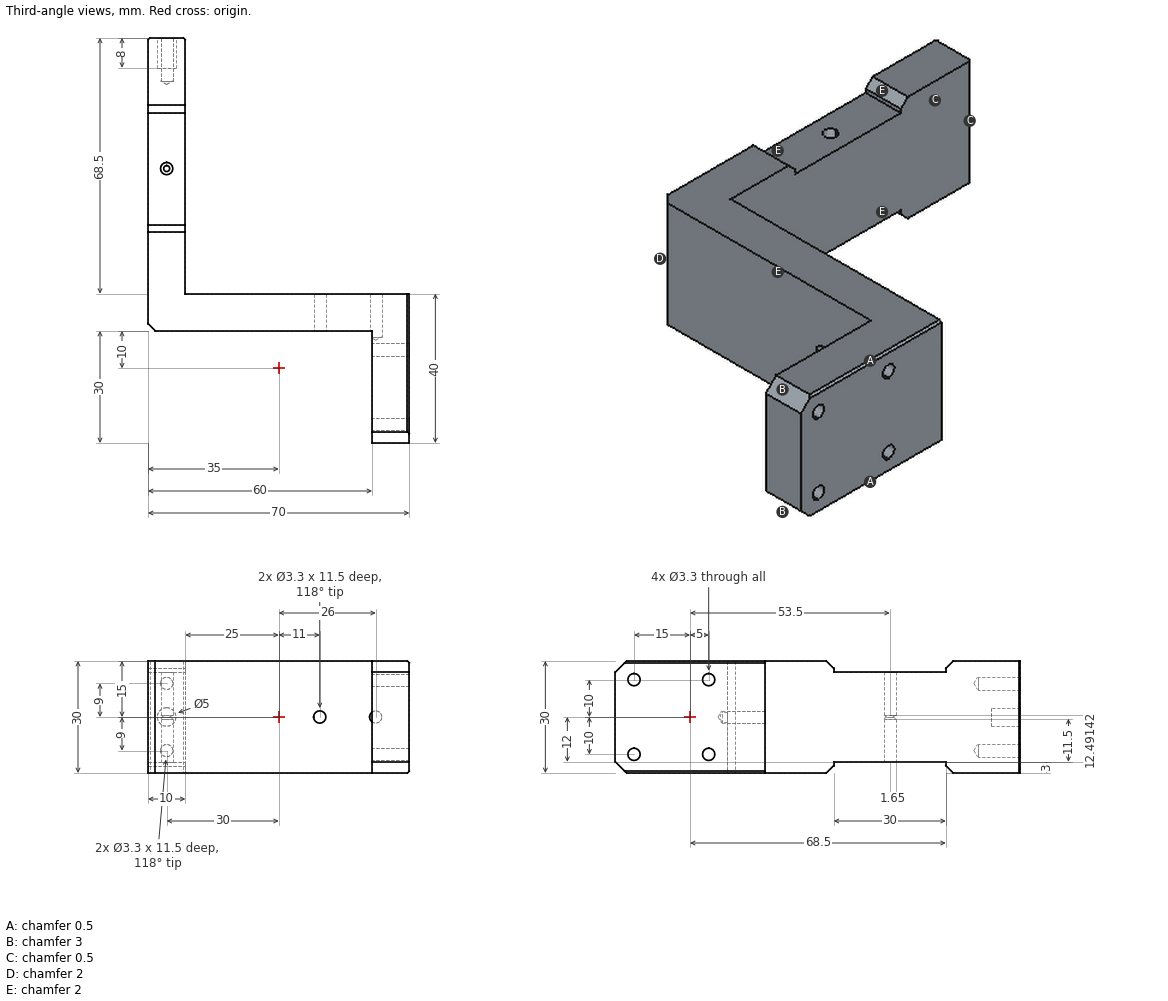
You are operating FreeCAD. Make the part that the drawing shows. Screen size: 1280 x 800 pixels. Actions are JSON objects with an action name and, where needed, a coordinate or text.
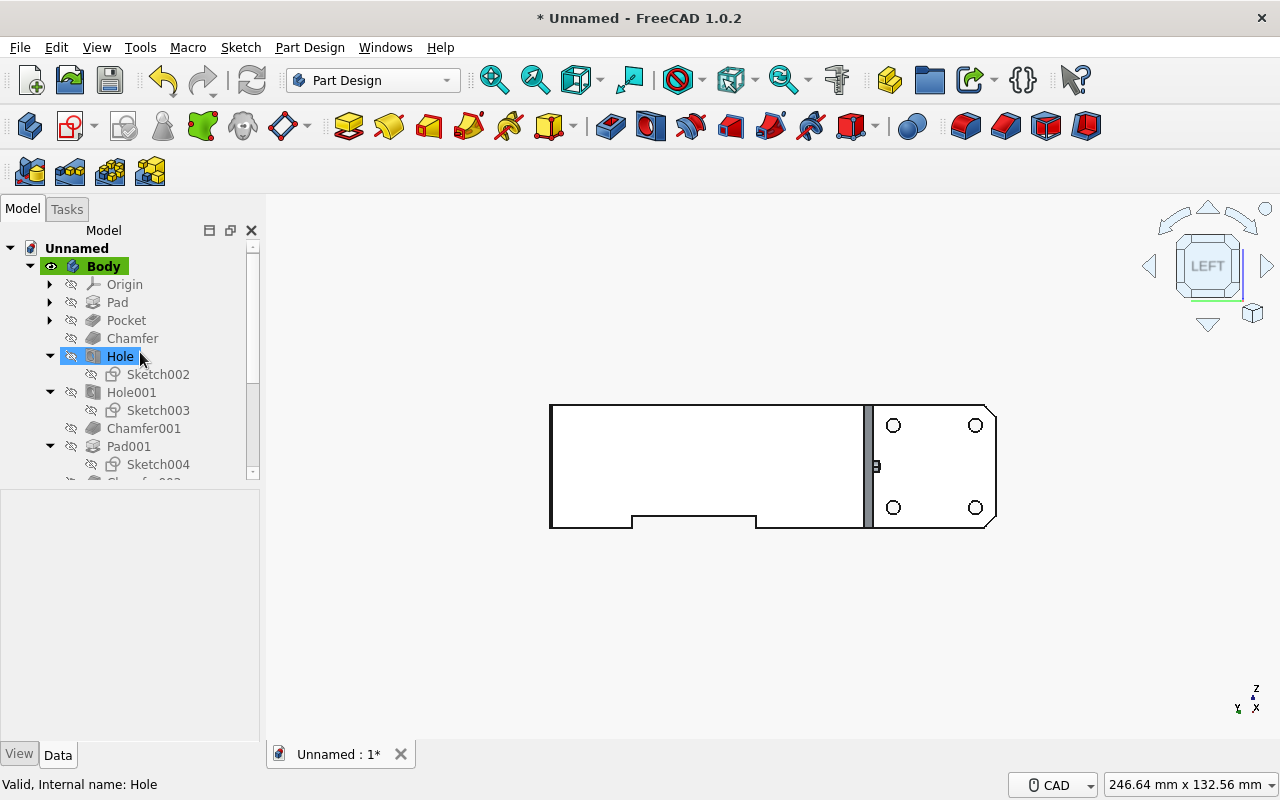
{"action": "left_click", "coordinate": [50, 284]}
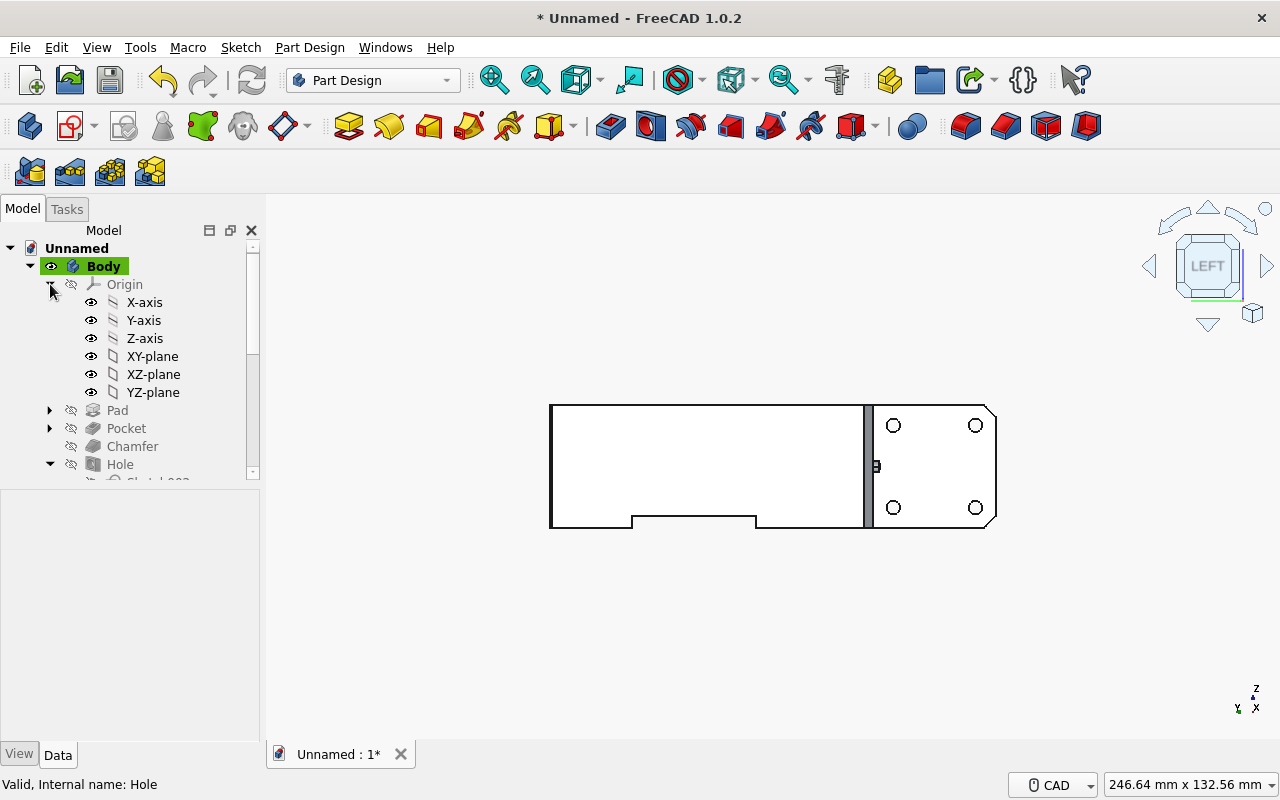
{"action": "left_click", "coordinate": [136, 392]}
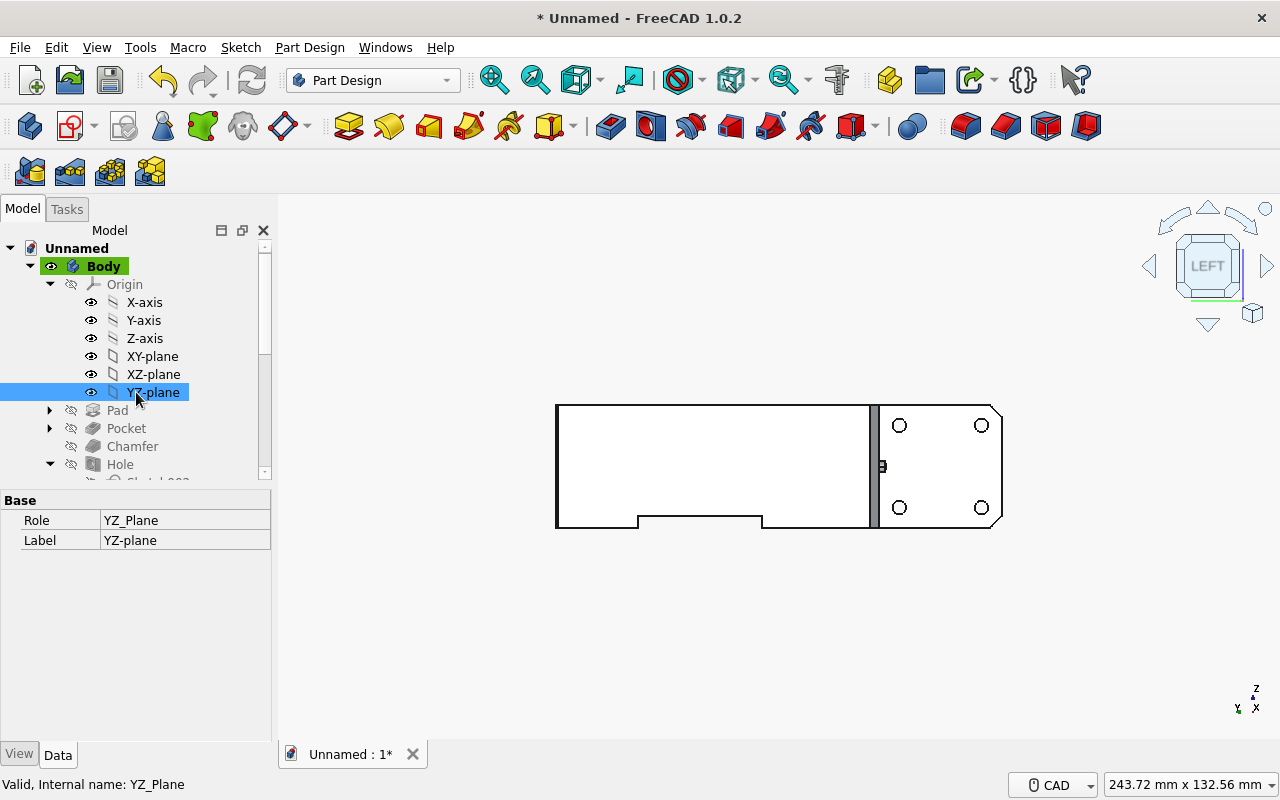
{"action": "left_click", "coordinate": [284, 126]}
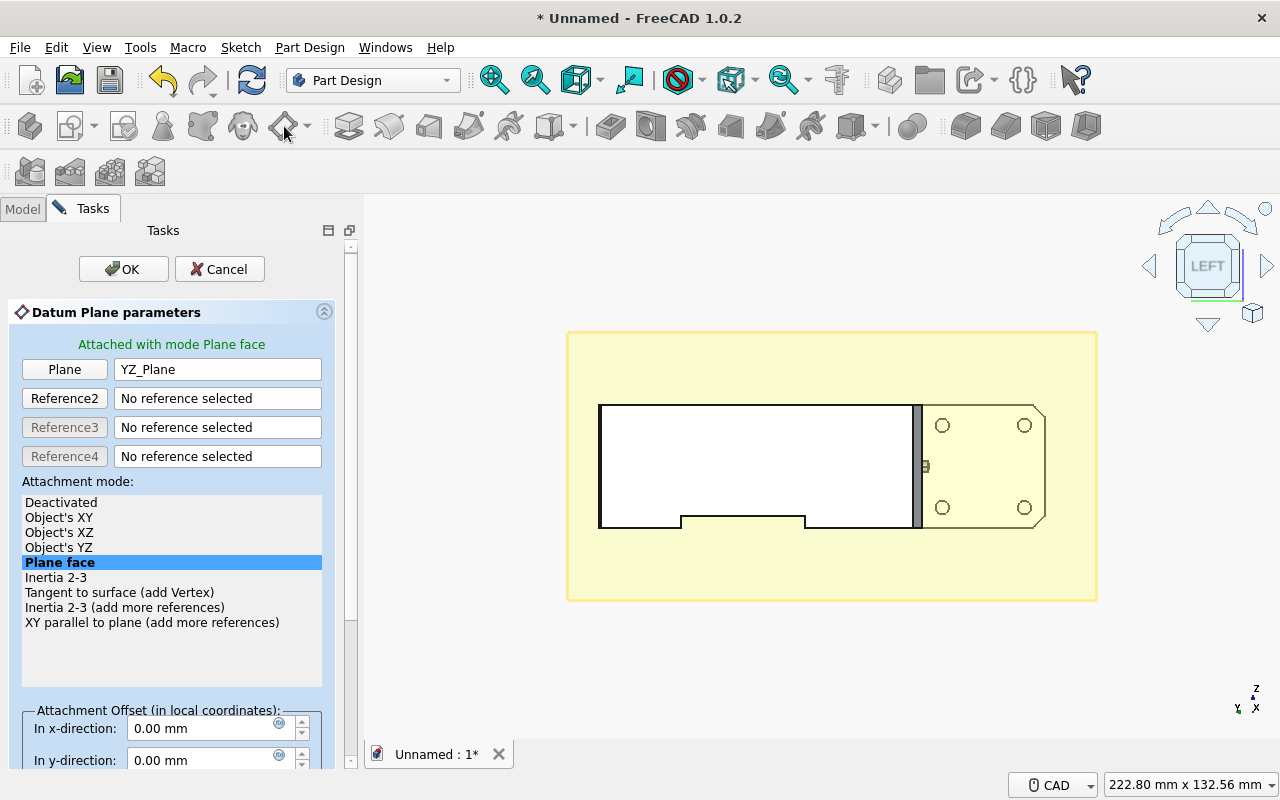
{"action": "scroll", "coordinate": [351, 504], "scroll_direction": "down", "scroll_amount": 2}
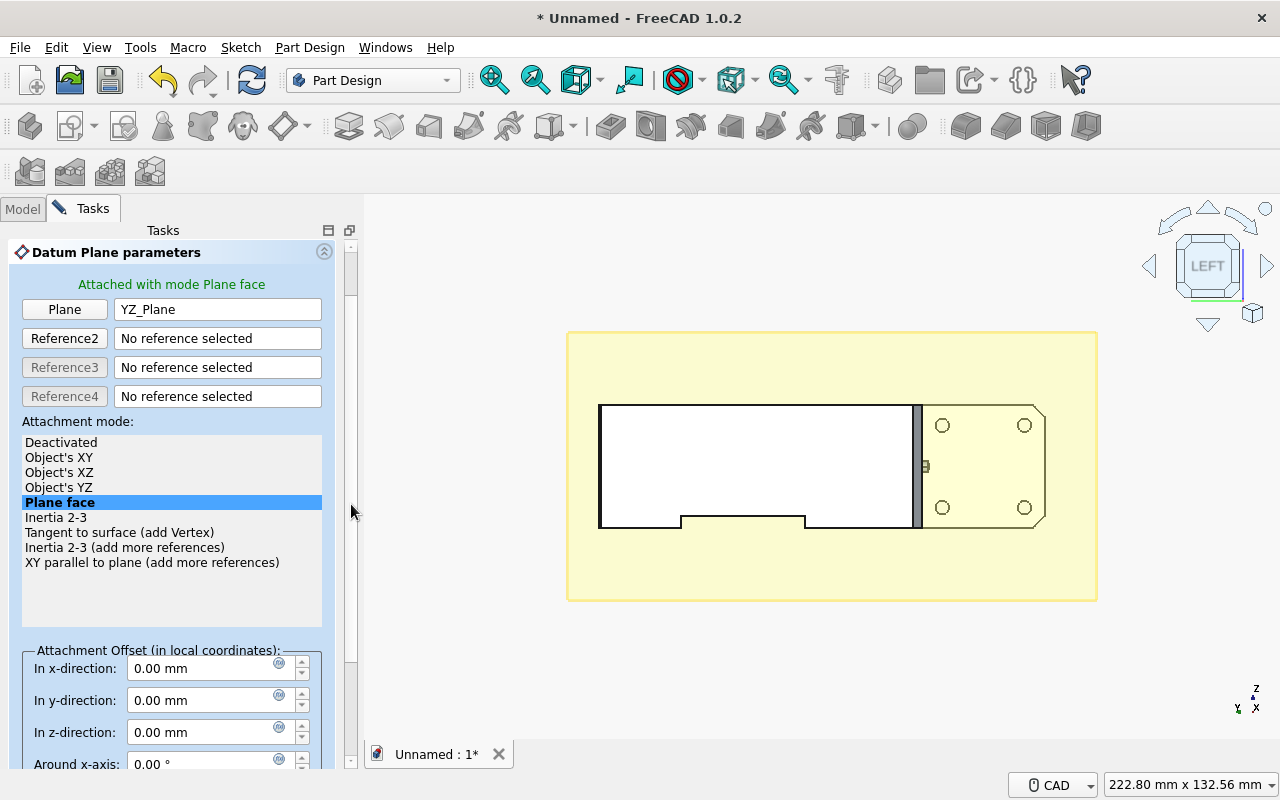
{"action": "triple_click", "coordinate": [210, 672]}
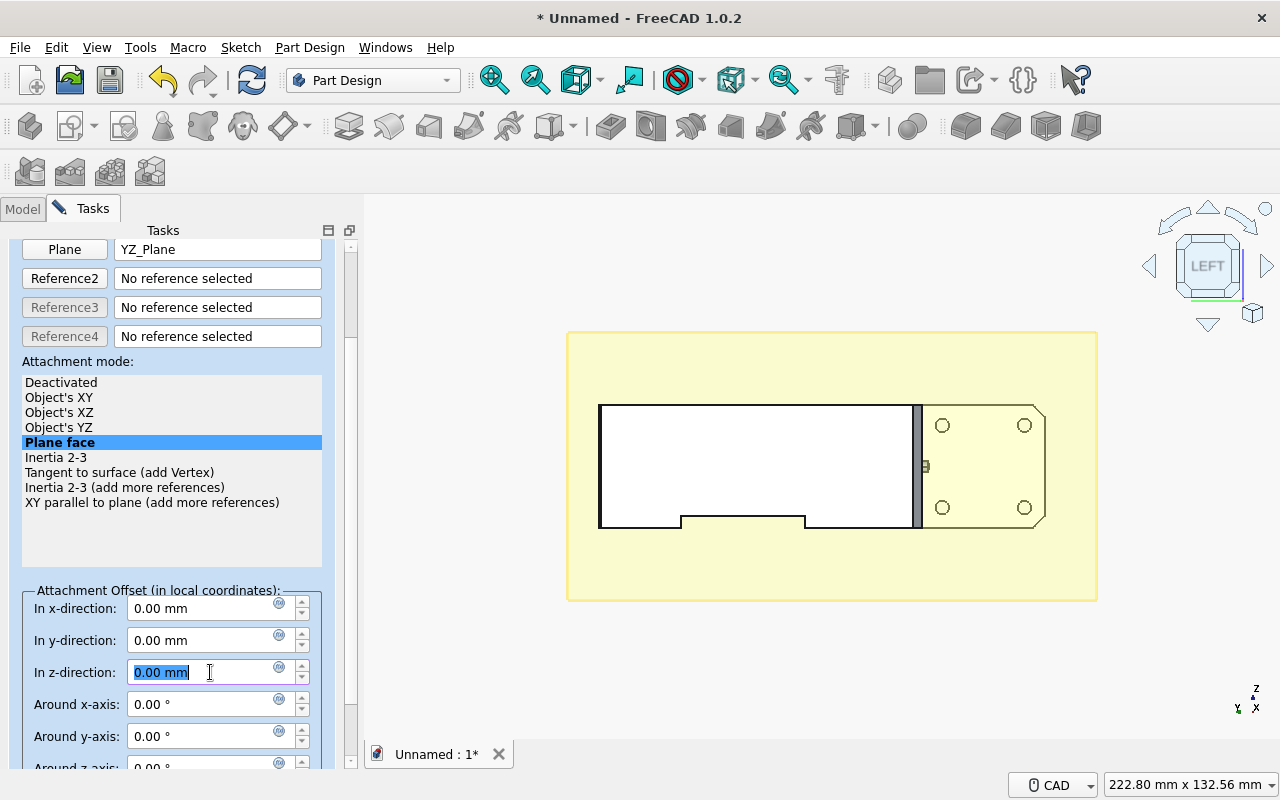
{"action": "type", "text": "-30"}
{"action": "key", "text": "Tab"}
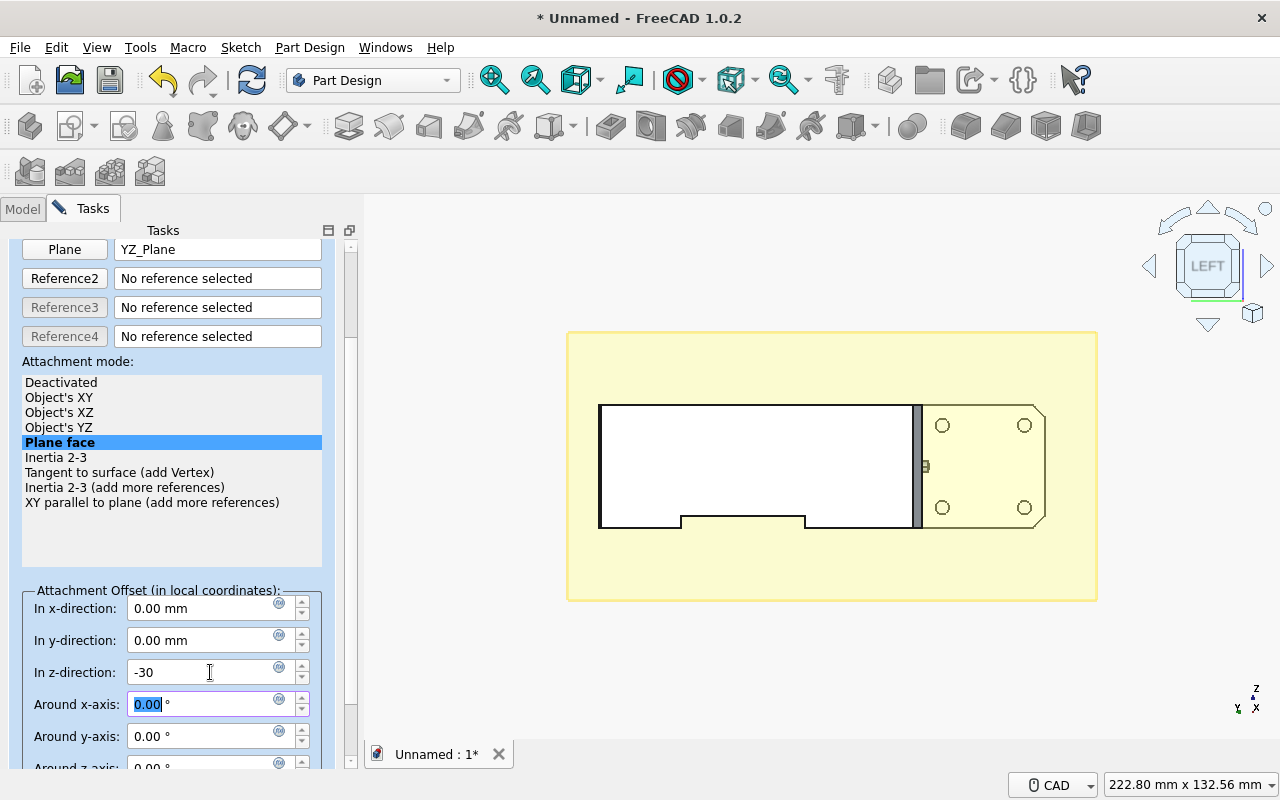
{"action": "scroll", "coordinate": [351, 504], "scroll_direction": "up", "scroll_amount": 3}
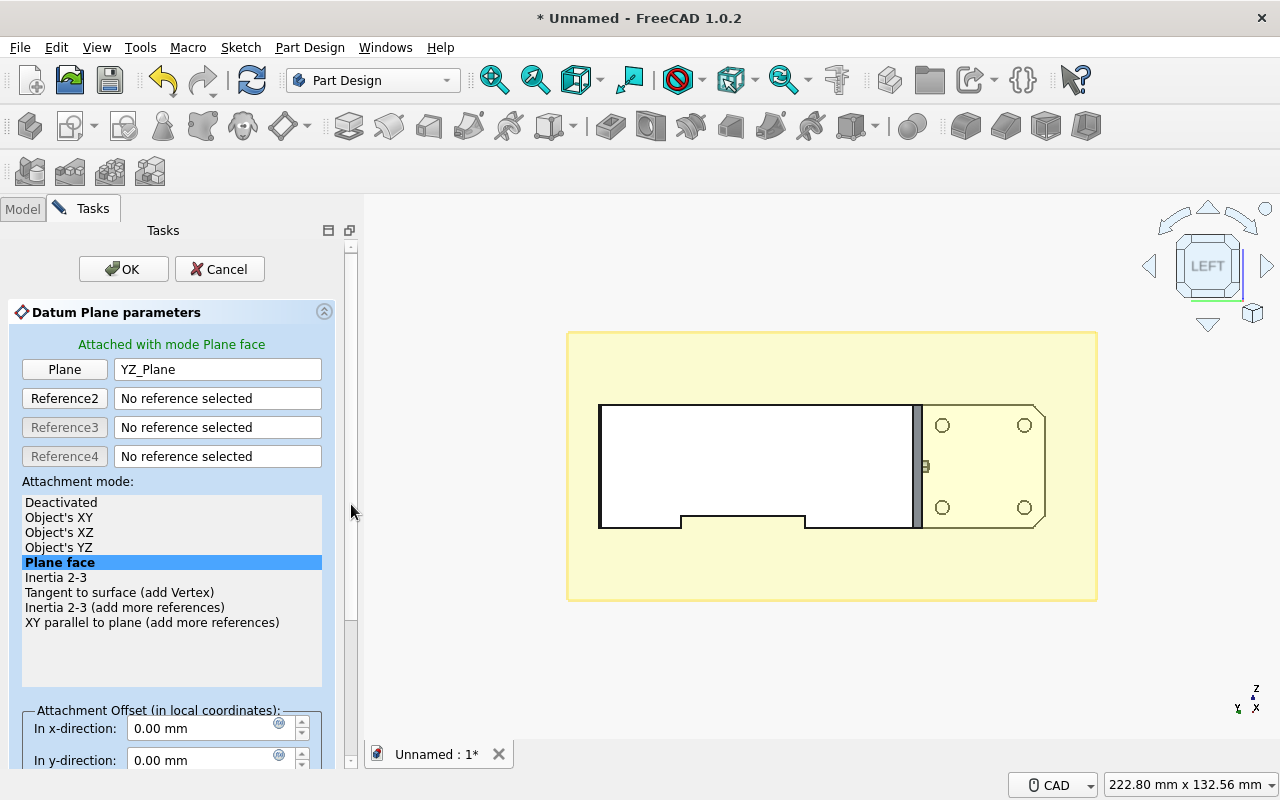
{"action": "left_click", "coordinate": [124, 269]}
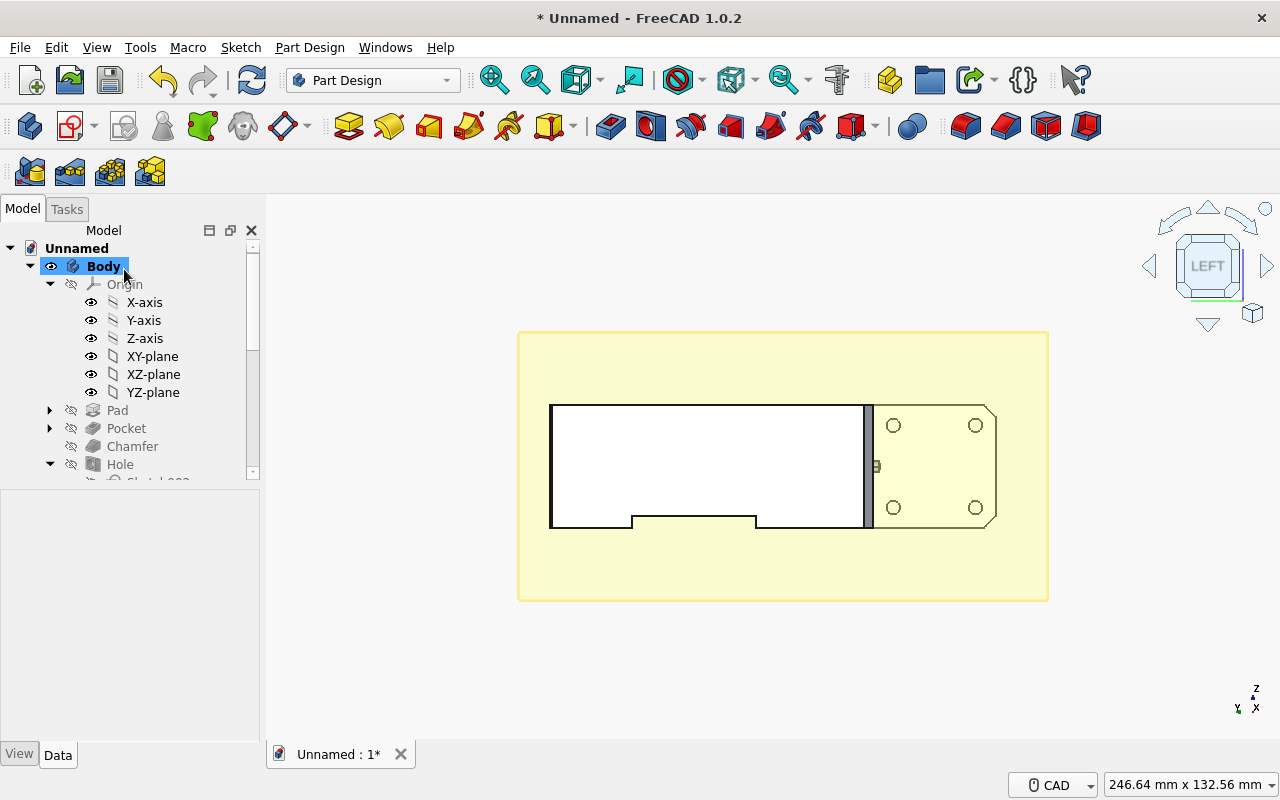
{"action": "scroll", "coordinate": [100, 352], "scroll_direction": "down", "scroll_amount": 3}